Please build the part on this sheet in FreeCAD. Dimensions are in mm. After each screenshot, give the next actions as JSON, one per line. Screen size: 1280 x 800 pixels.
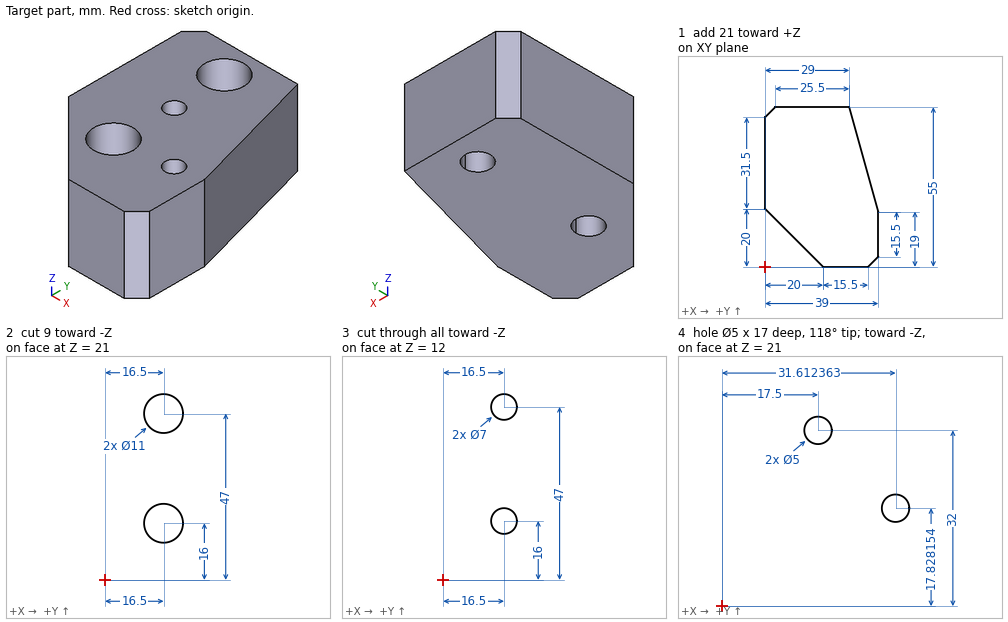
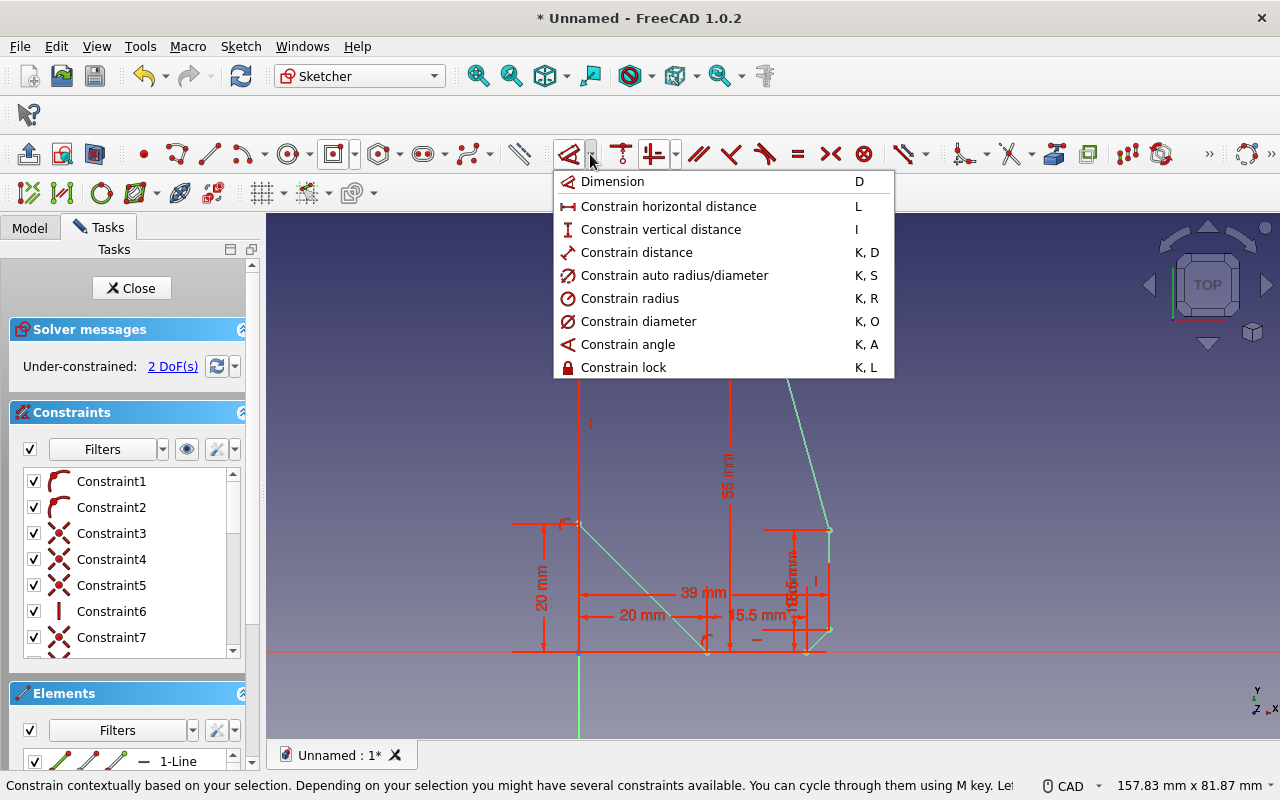
{"action": "left_click", "coordinate": [724, 206]}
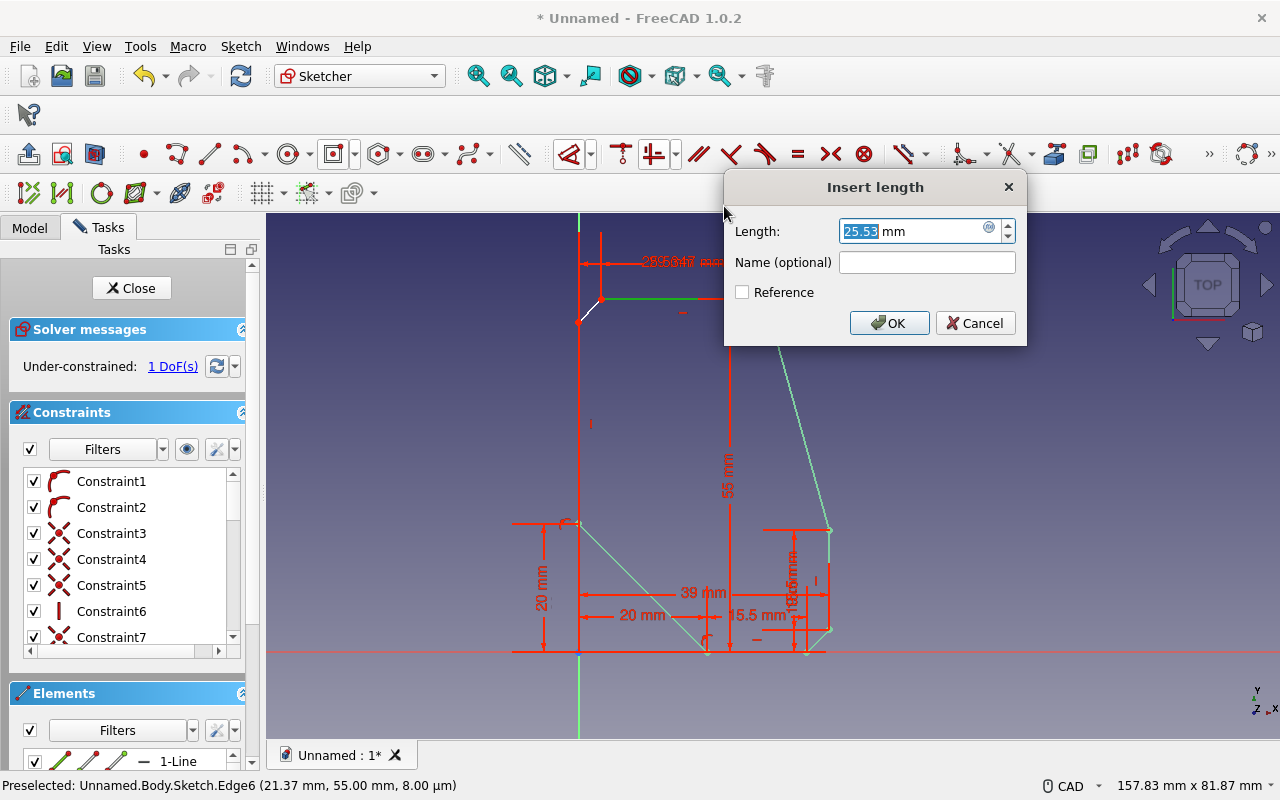
{"action": "type", "text": "25.5"}
{"action": "key", "text": "Return"}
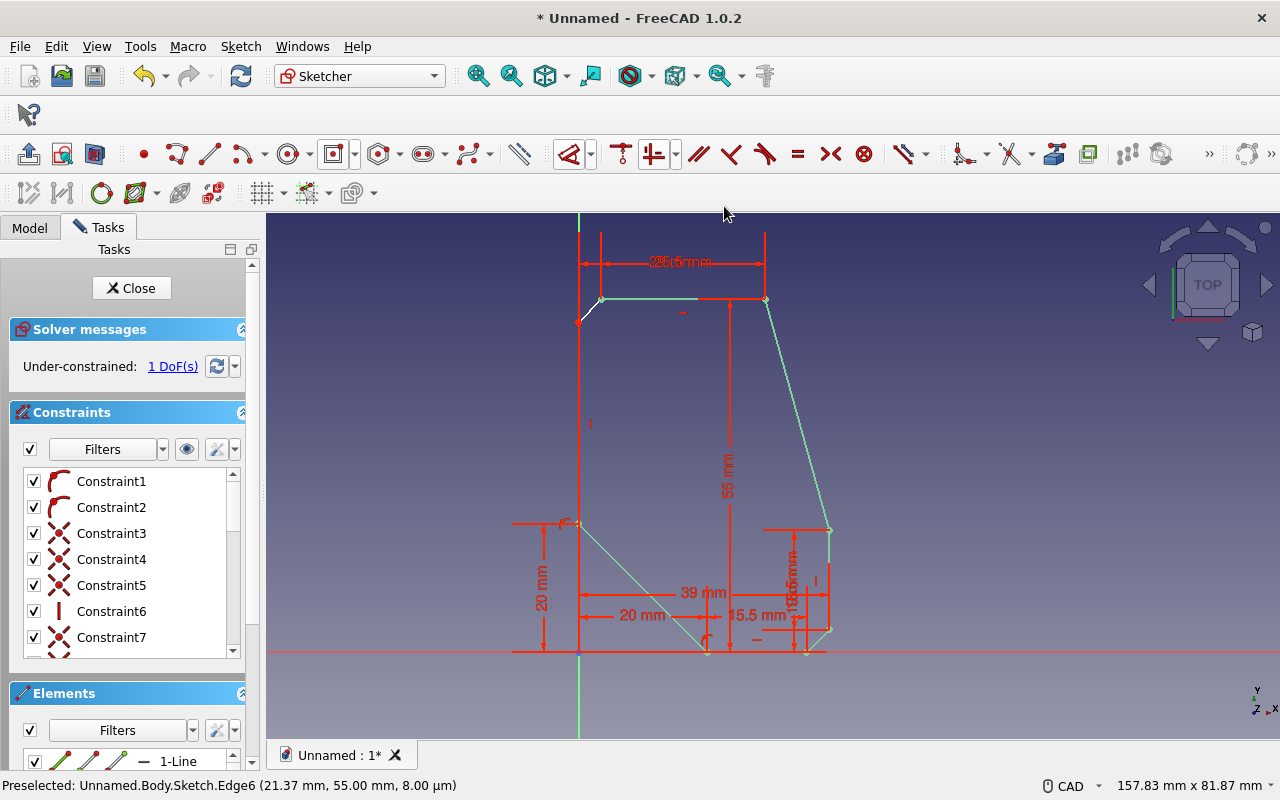
{"action": "left_click", "coordinate": [579, 383]}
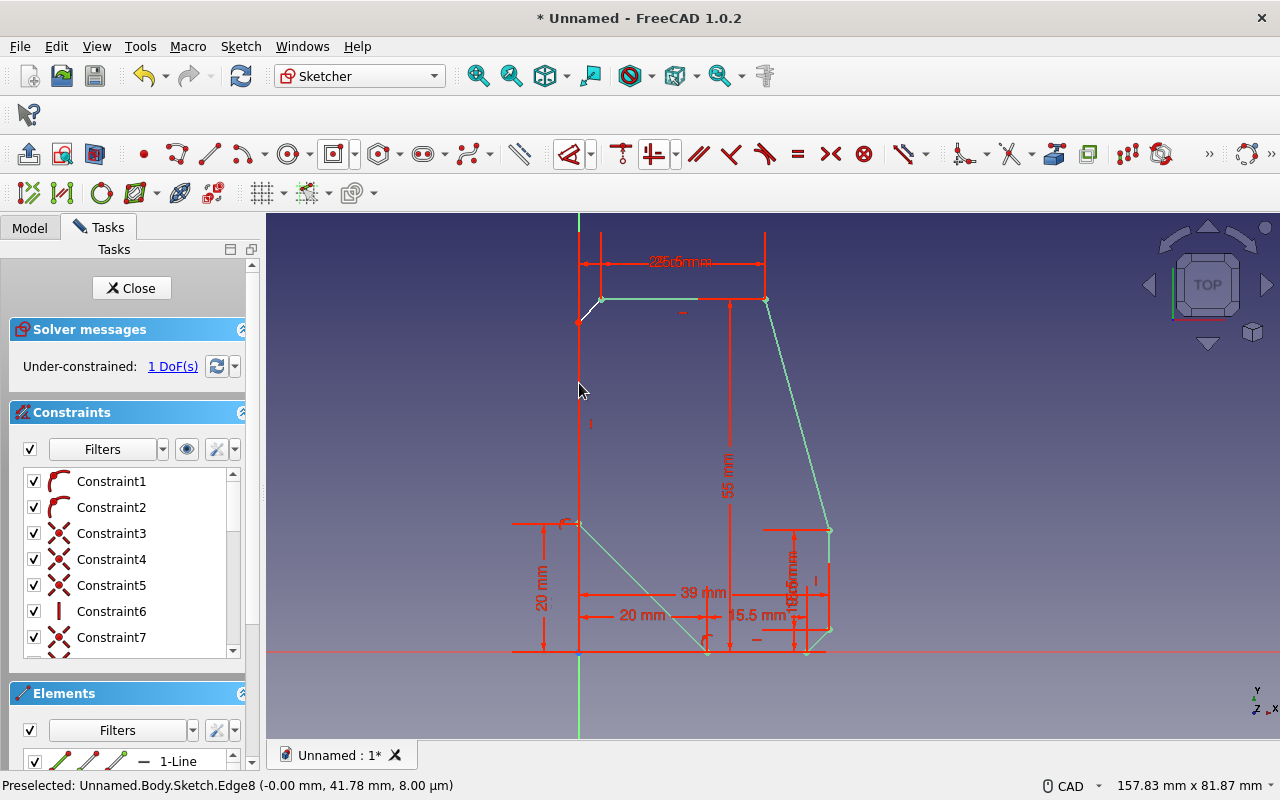
{"action": "left_click", "coordinate": [590, 154]}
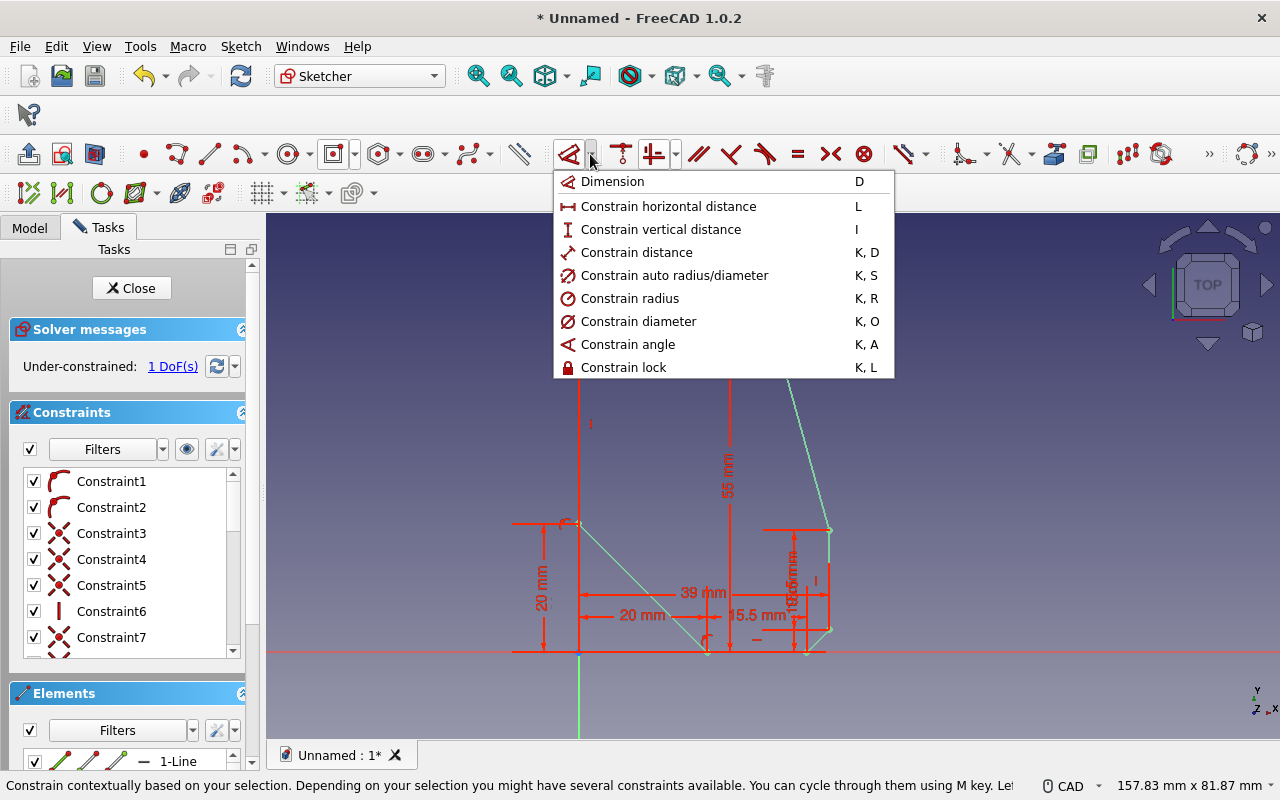
{"action": "left_click", "coordinate": [724, 230]}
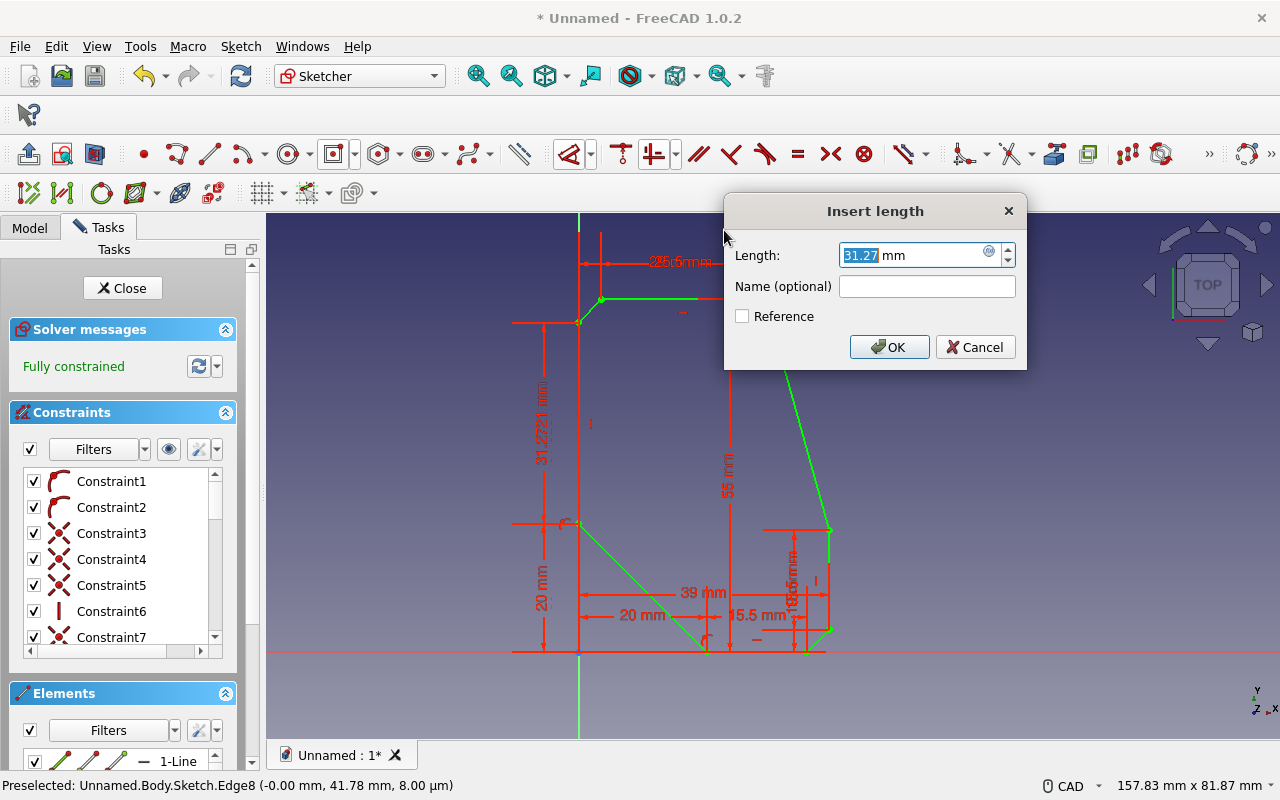
{"action": "type", "text": "31.5"}
{"action": "key", "text": "Return"}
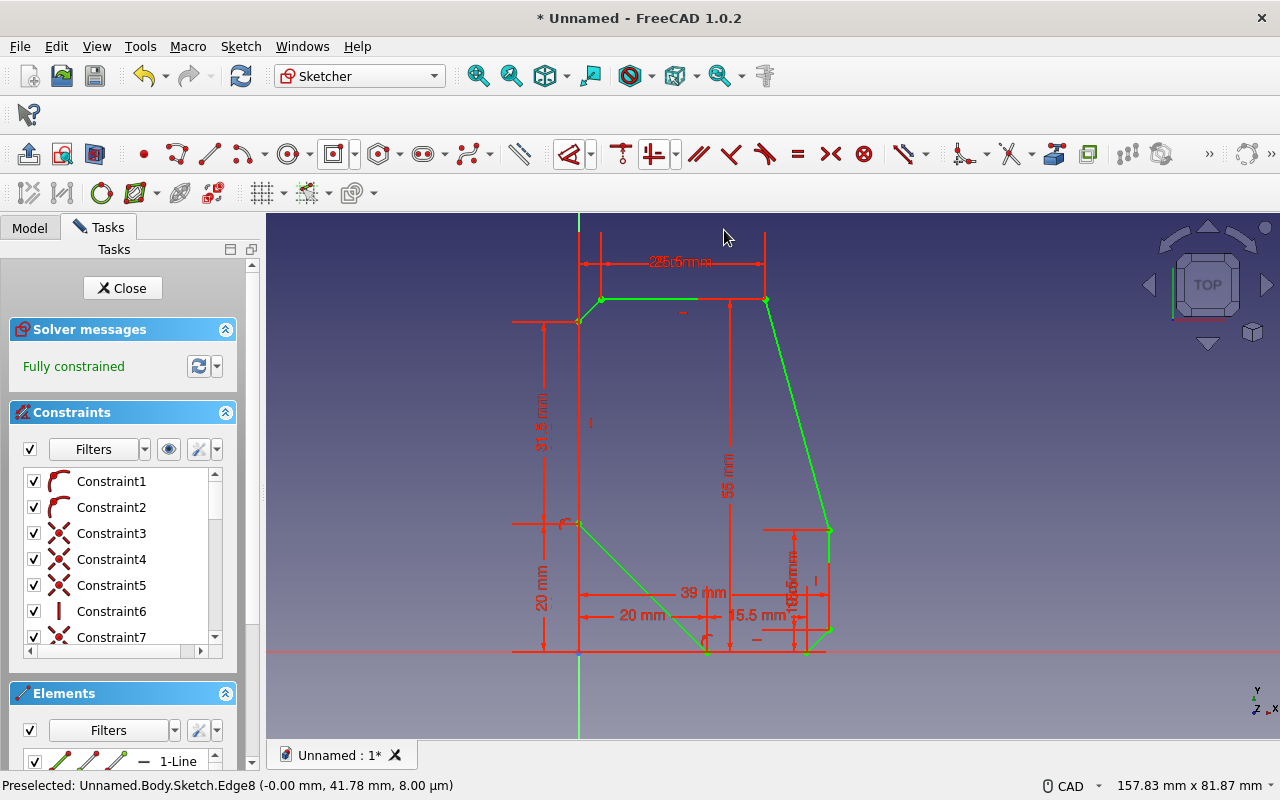
{"action": "left_click", "coordinate": [123, 288]}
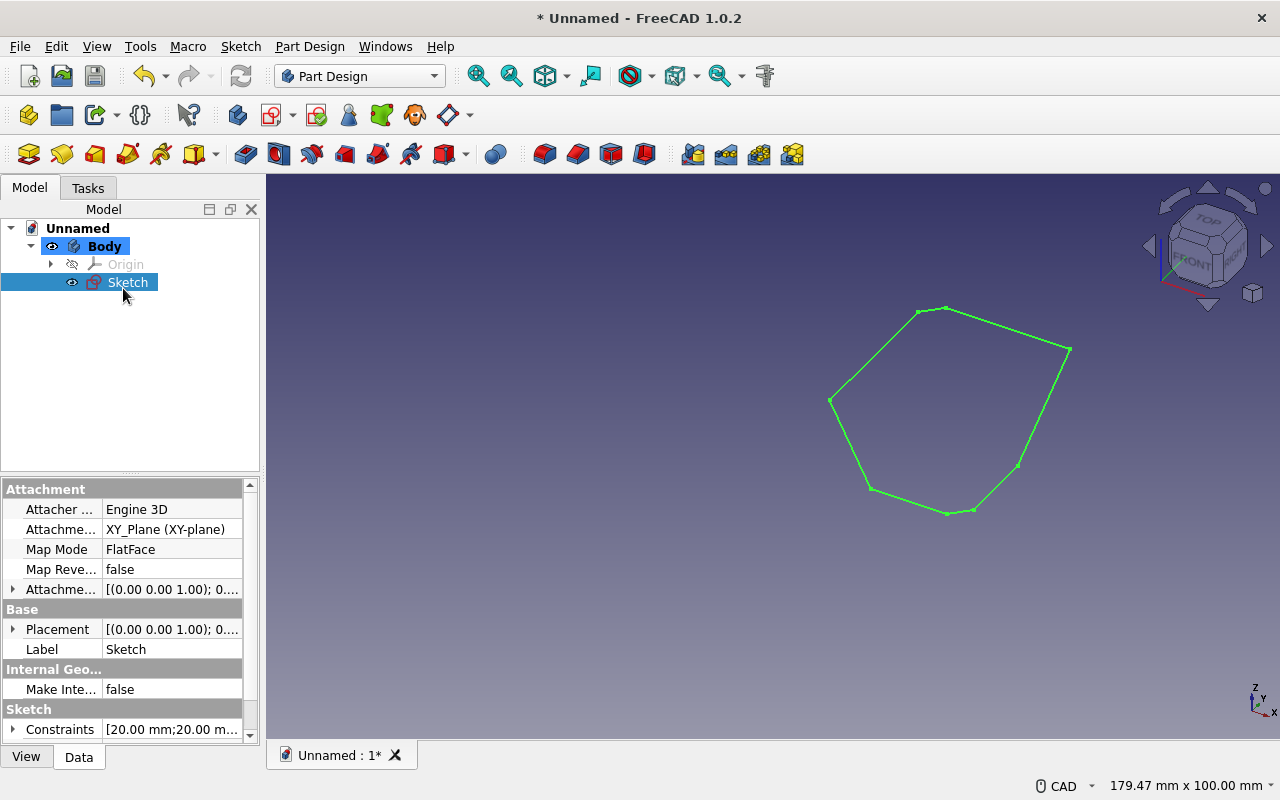
{"action": "left_click", "coordinate": [29, 154]}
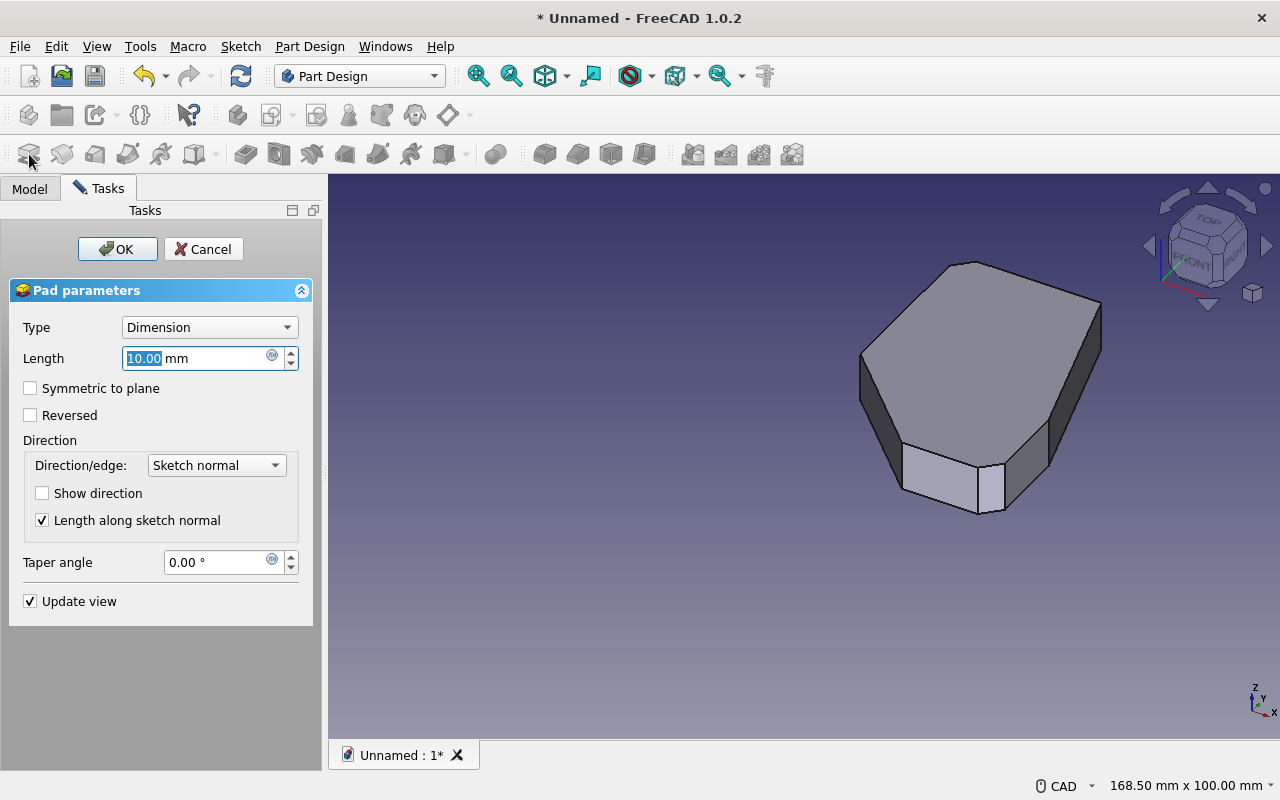
{"action": "type", "text": "21"}
{"action": "key", "text": "Tab"}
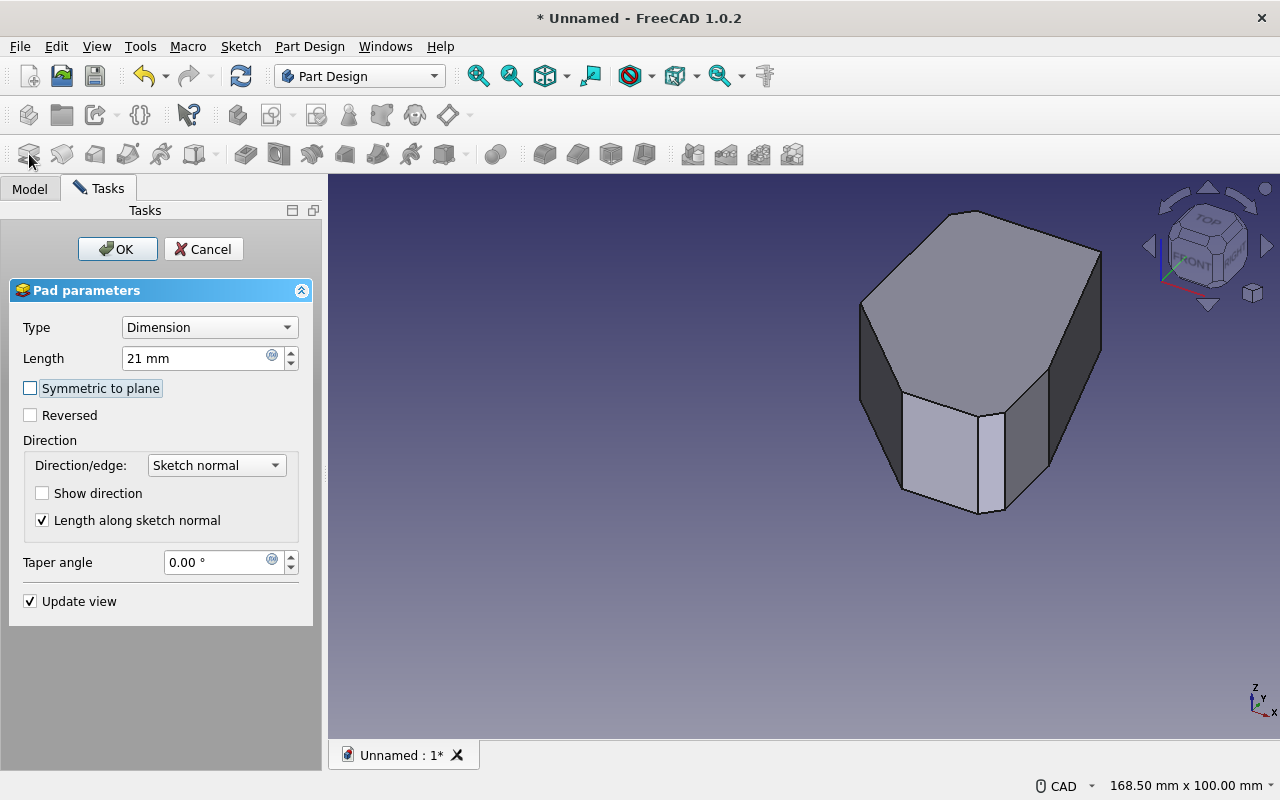
{"action": "left_click", "coordinate": [118, 249]}